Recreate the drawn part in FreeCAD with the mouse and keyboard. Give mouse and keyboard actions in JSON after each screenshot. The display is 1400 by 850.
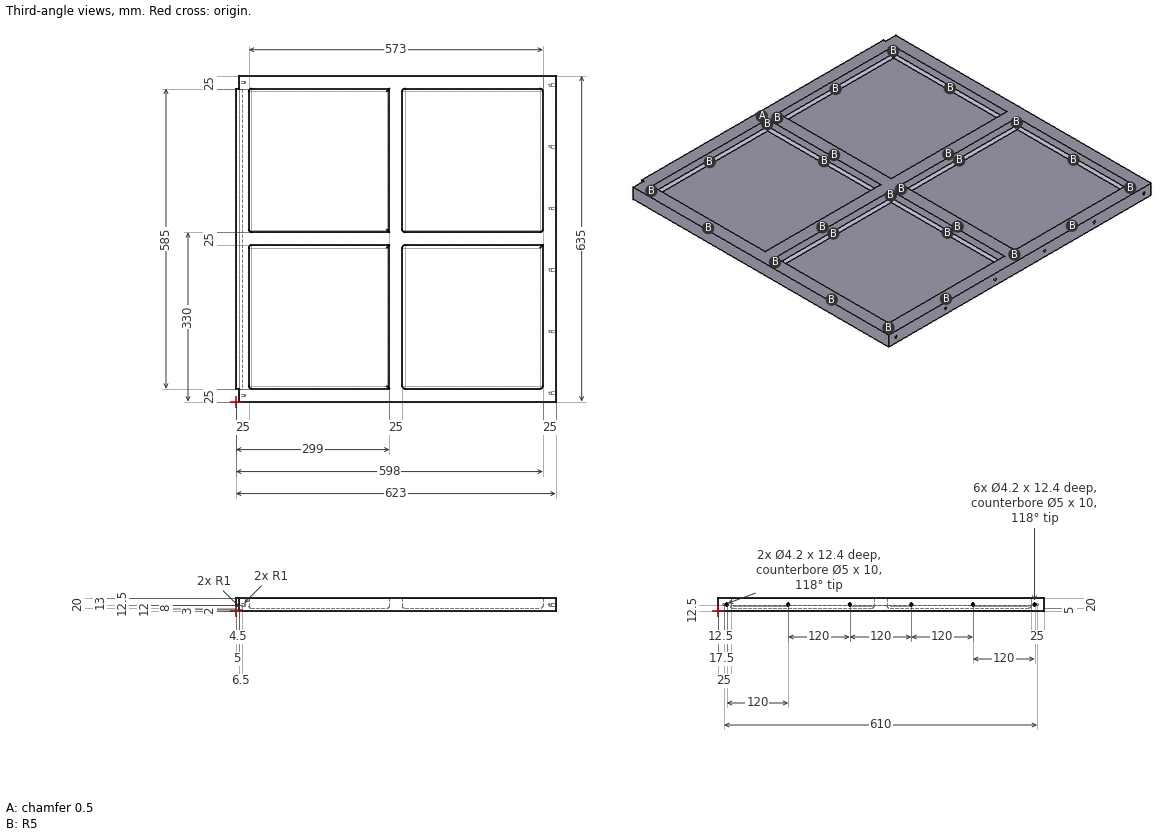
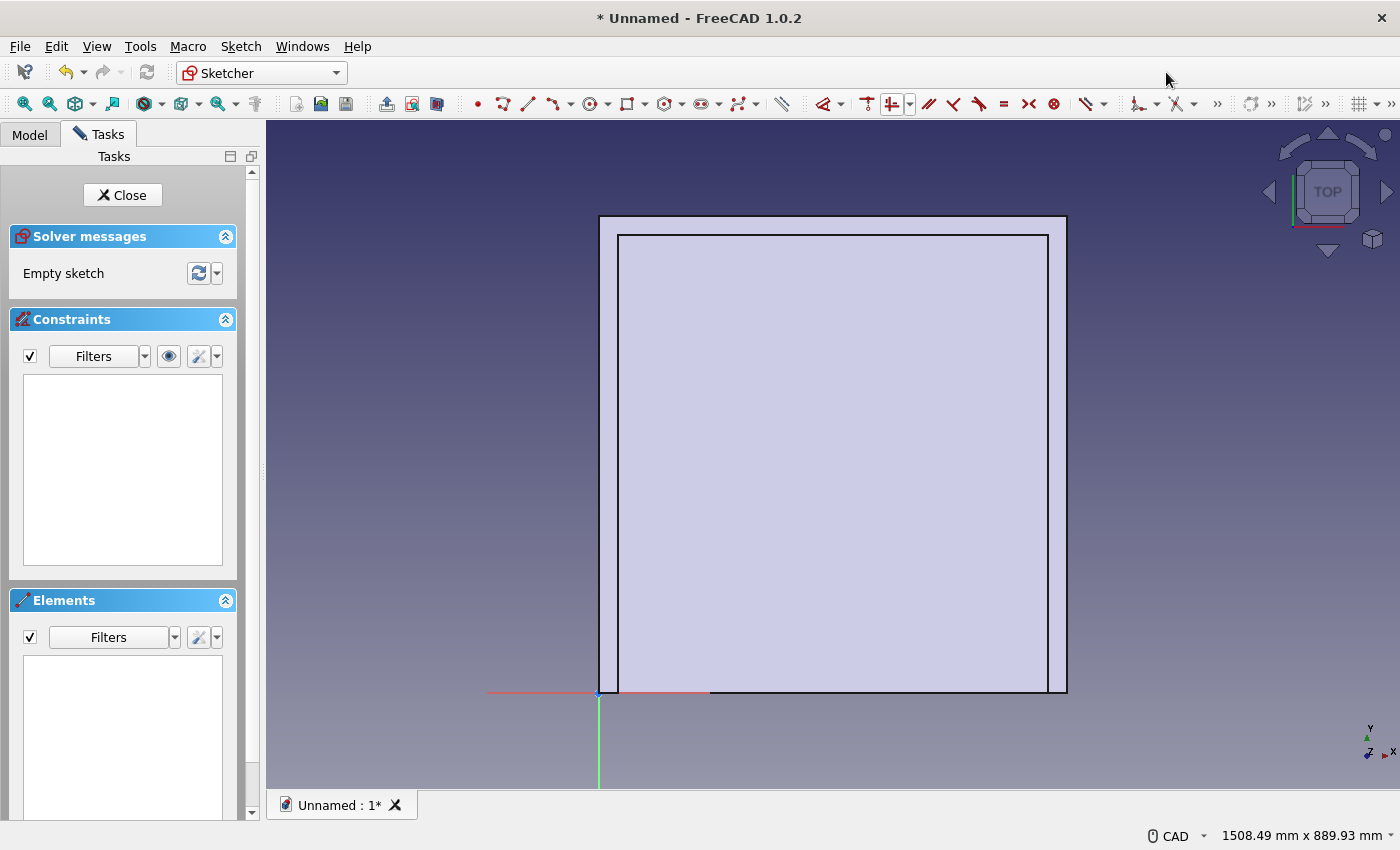
{"action": "left_click", "coordinate": [437, 104]}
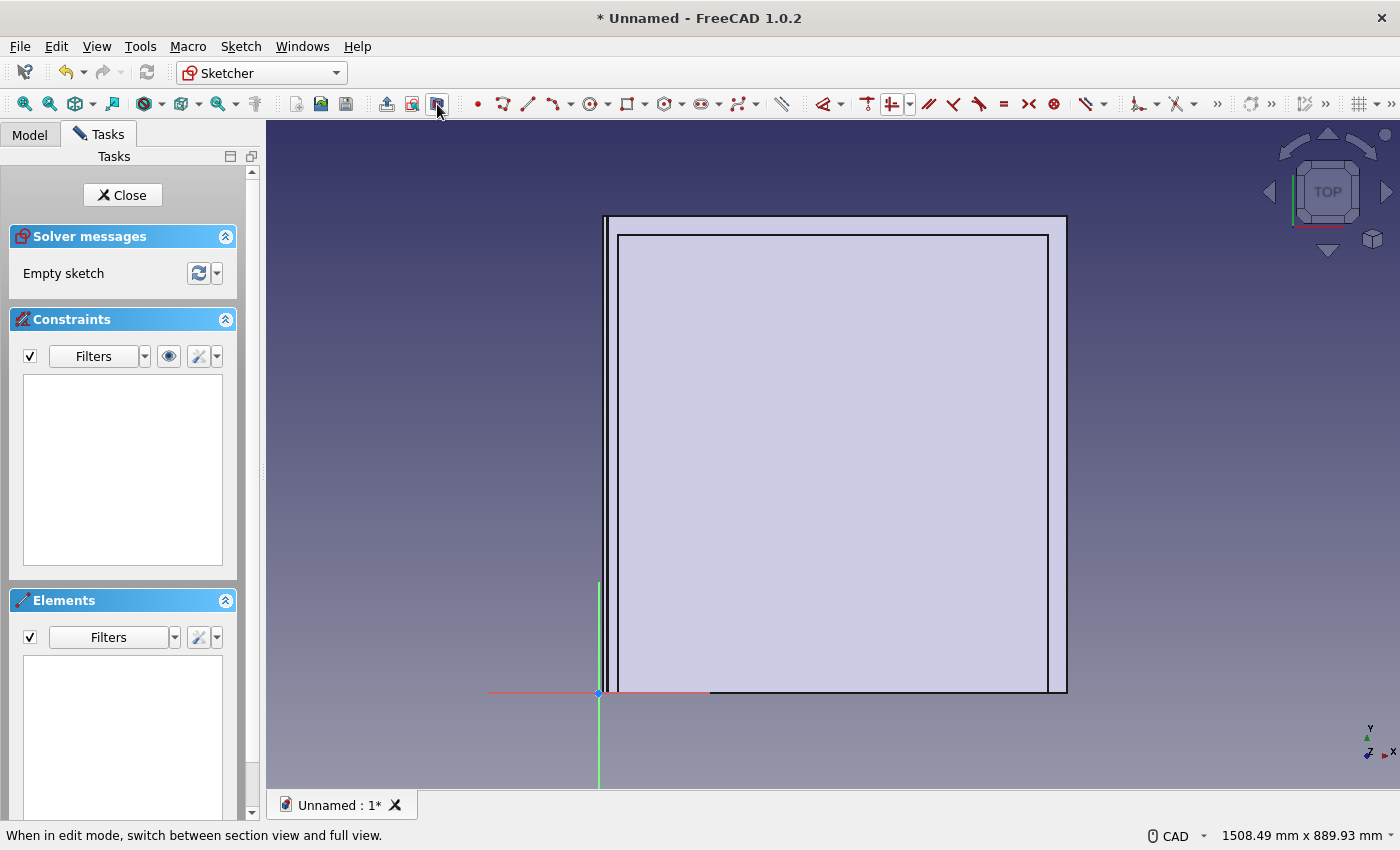
{"action": "scroll", "coordinate": [944, 761], "scroll_direction": "up", "scroll_amount": 2}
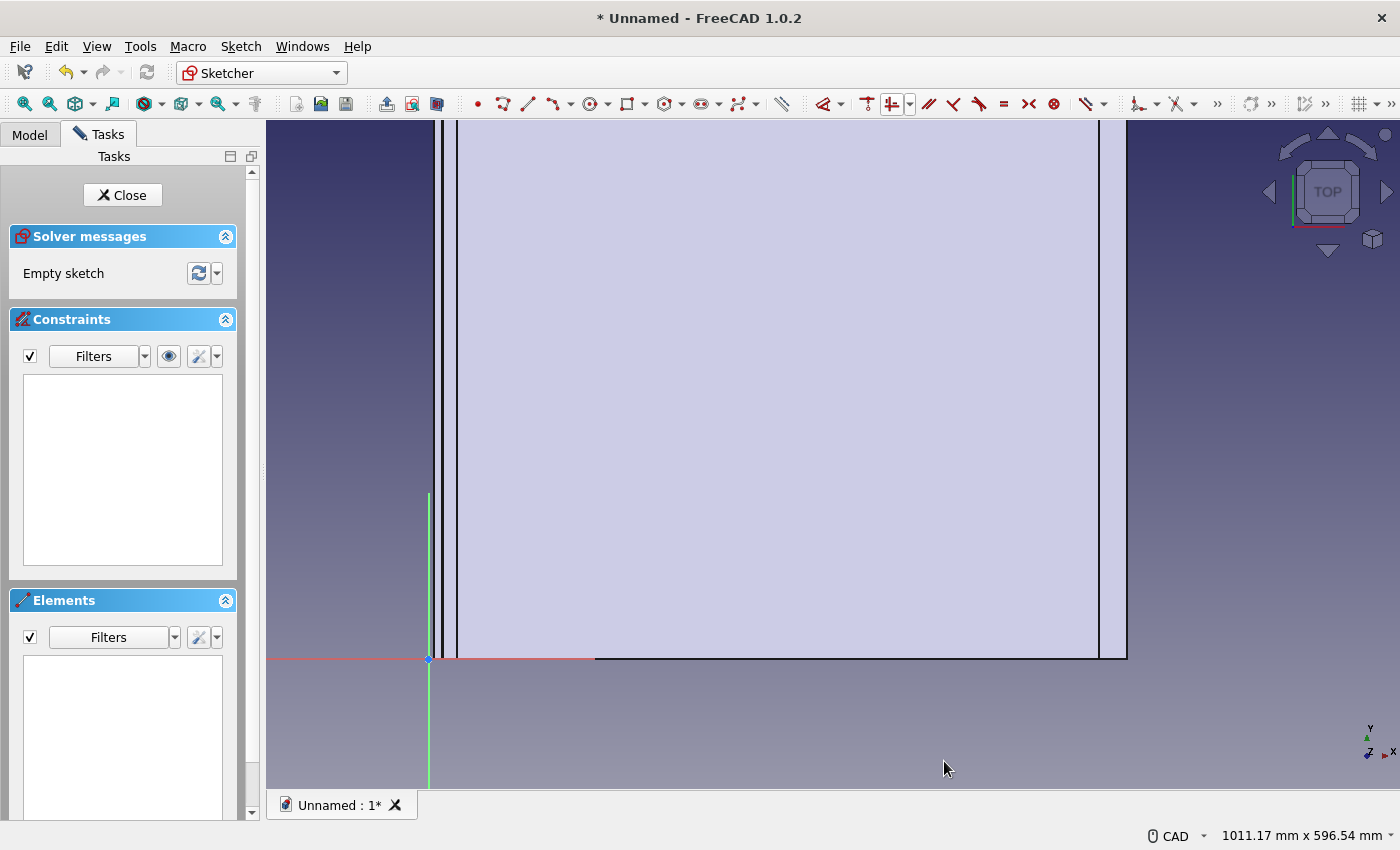
{"action": "left_click", "coordinate": [626, 104]}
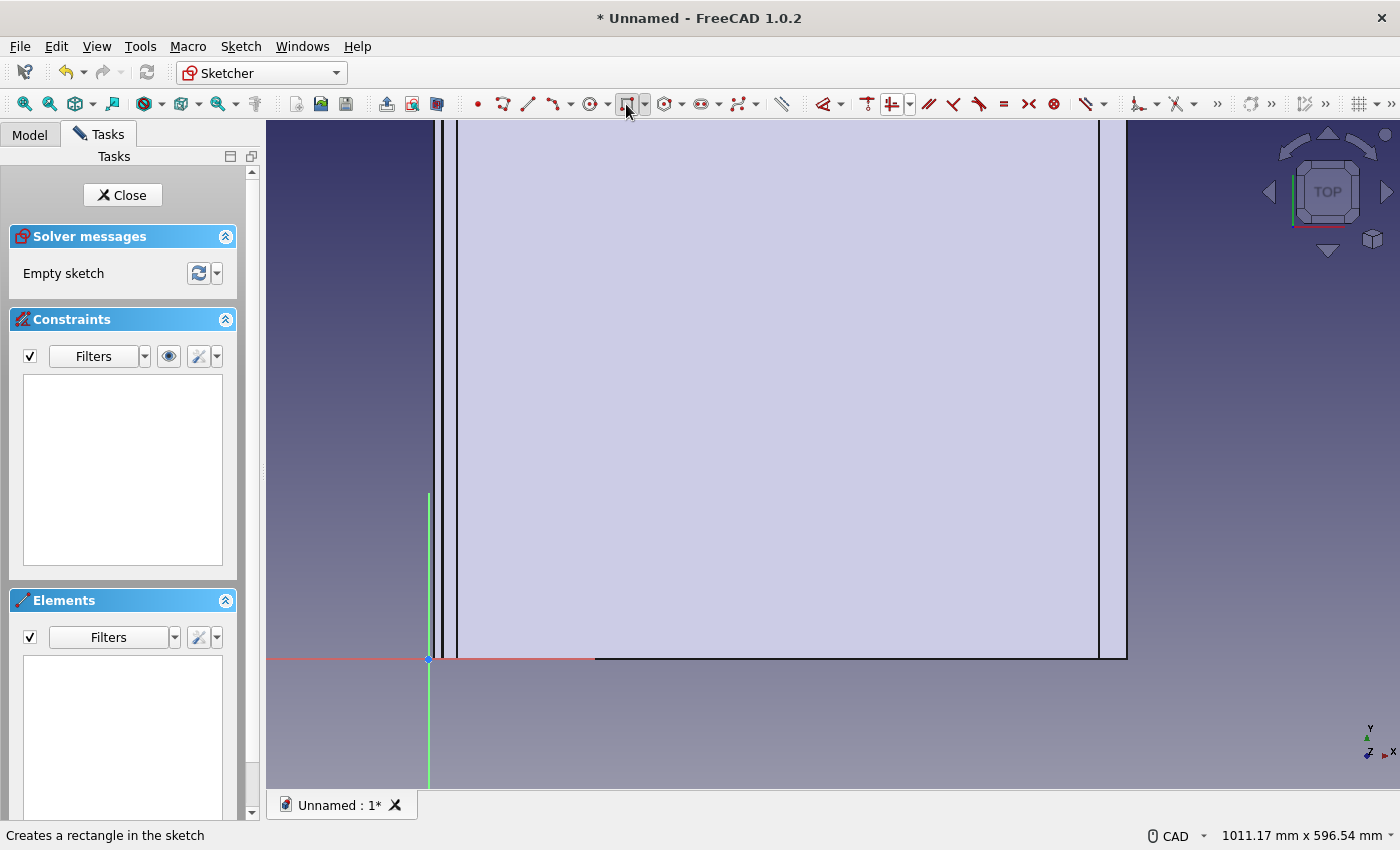
{"action": "left_click", "coordinate": [457, 631]}
{"action": "left_click", "coordinate": [1099, 659]}
{"action": "key", "text": "Escape"}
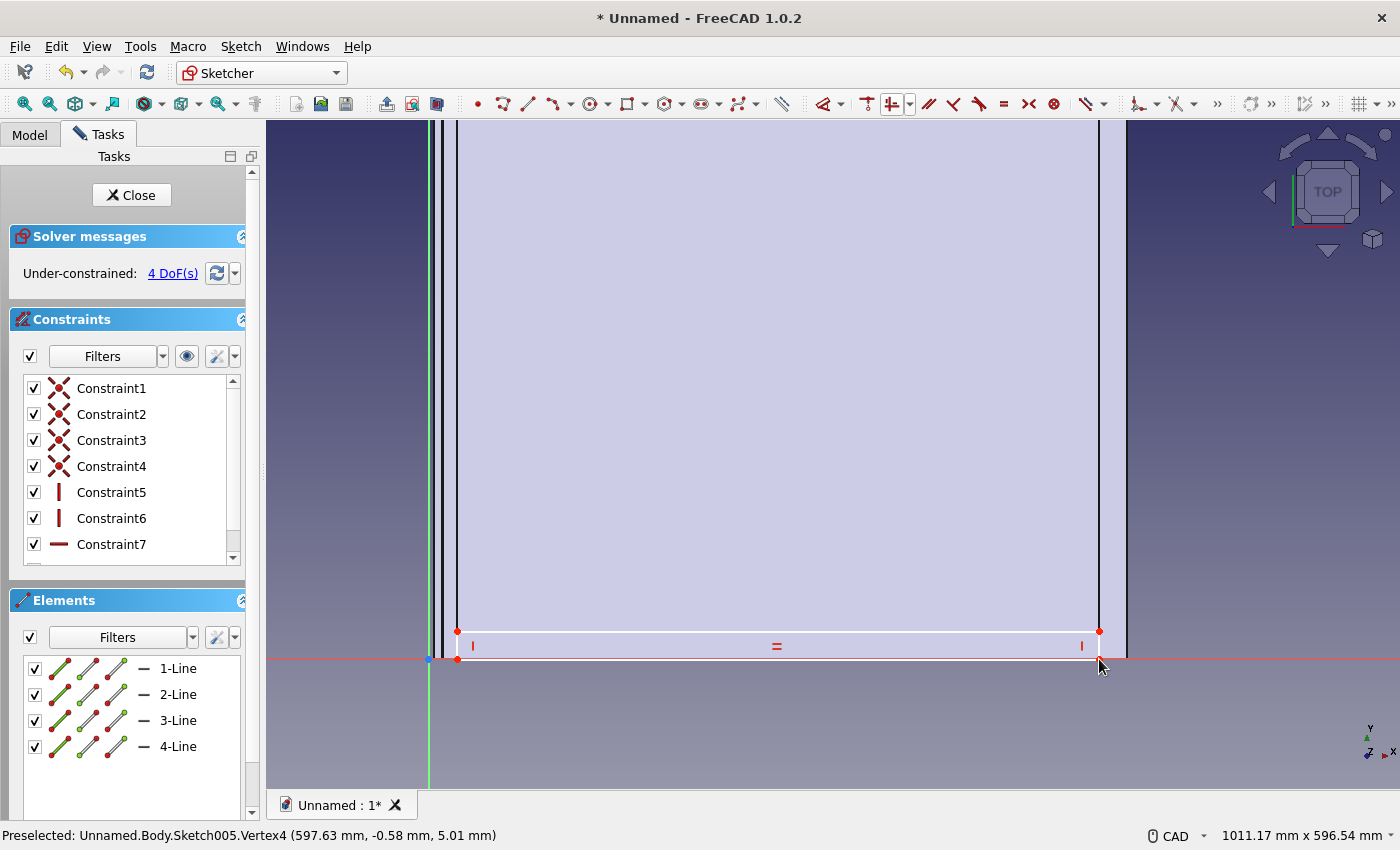
{"action": "left_click", "coordinate": [457, 660]}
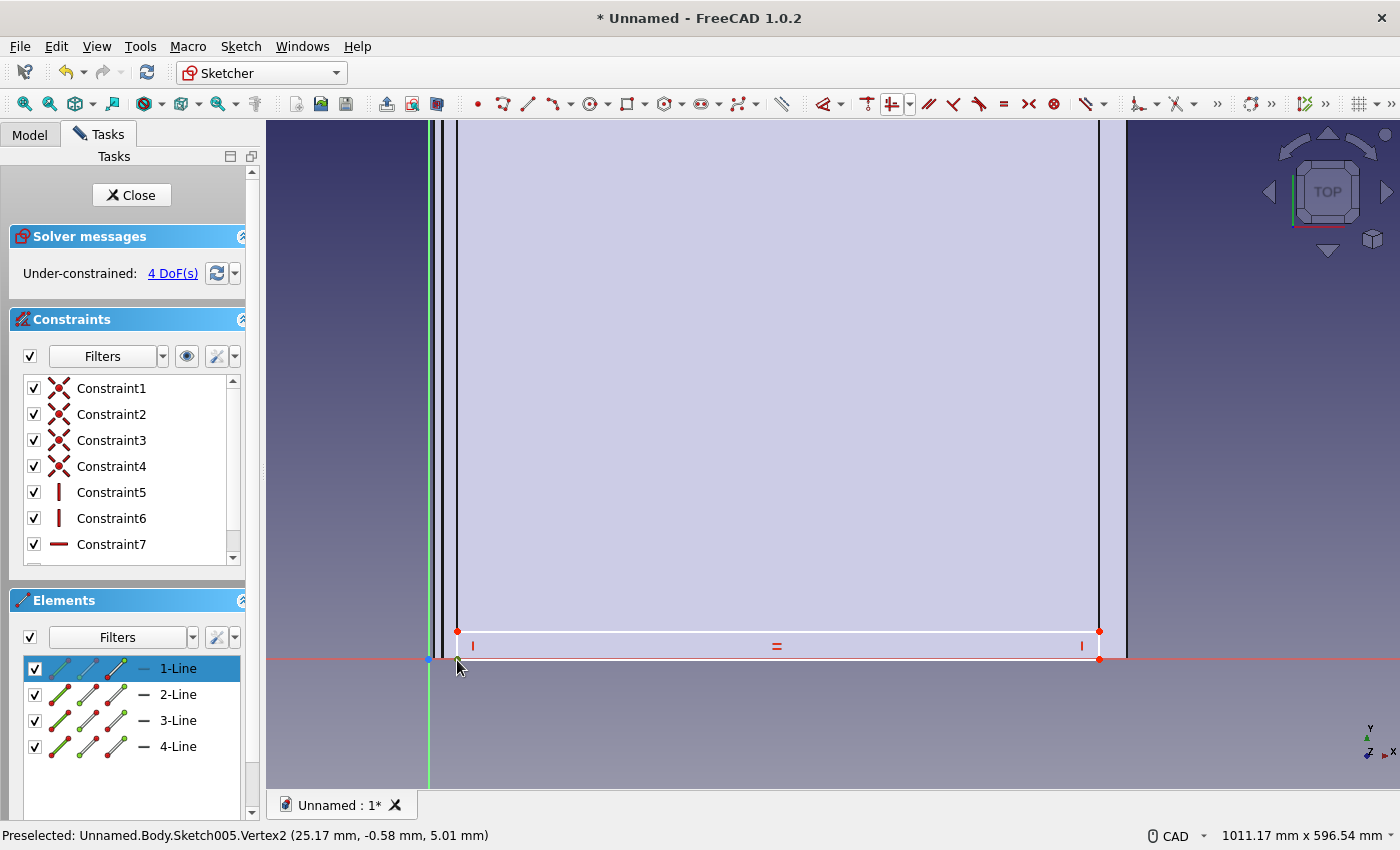
{"action": "left_click", "coordinate": [361, 659]}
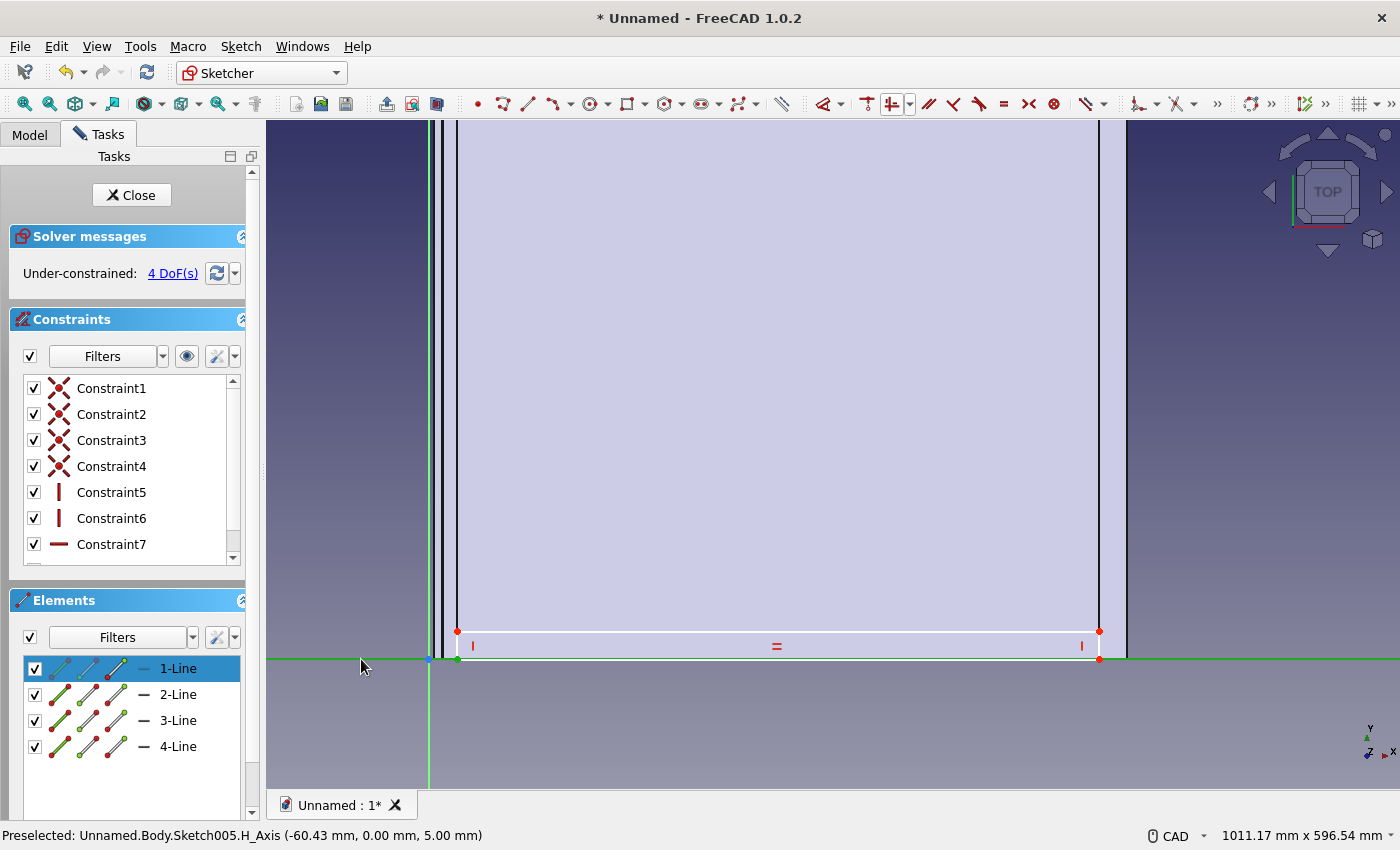
{"action": "left_click", "coordinate": [867, 104]}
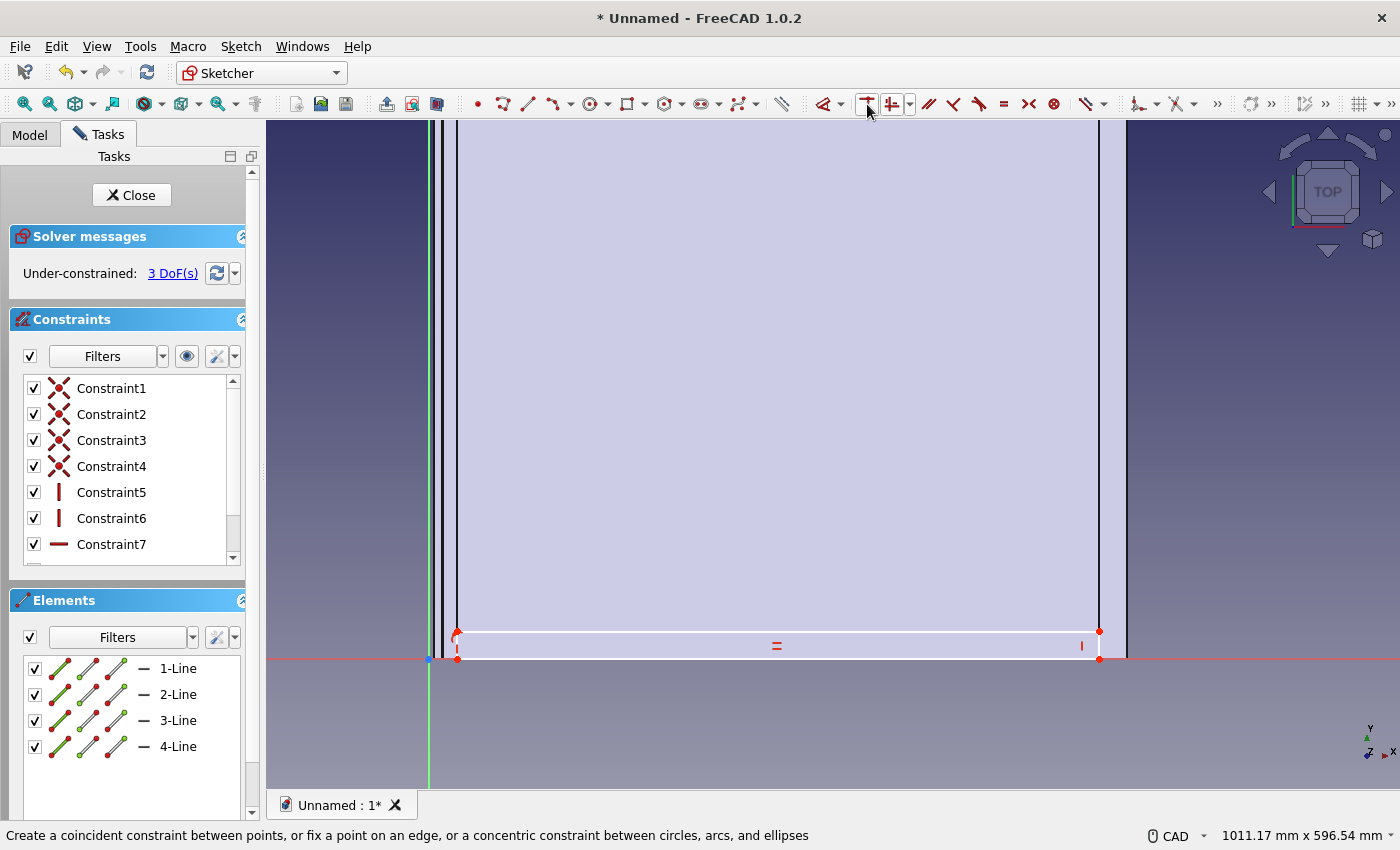
{"action": "left_click", "coordinate": [822, 104]}